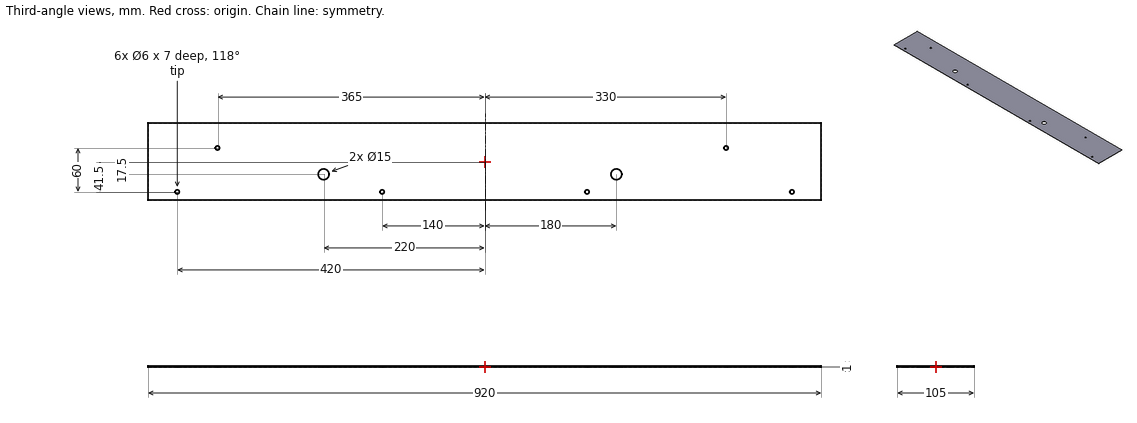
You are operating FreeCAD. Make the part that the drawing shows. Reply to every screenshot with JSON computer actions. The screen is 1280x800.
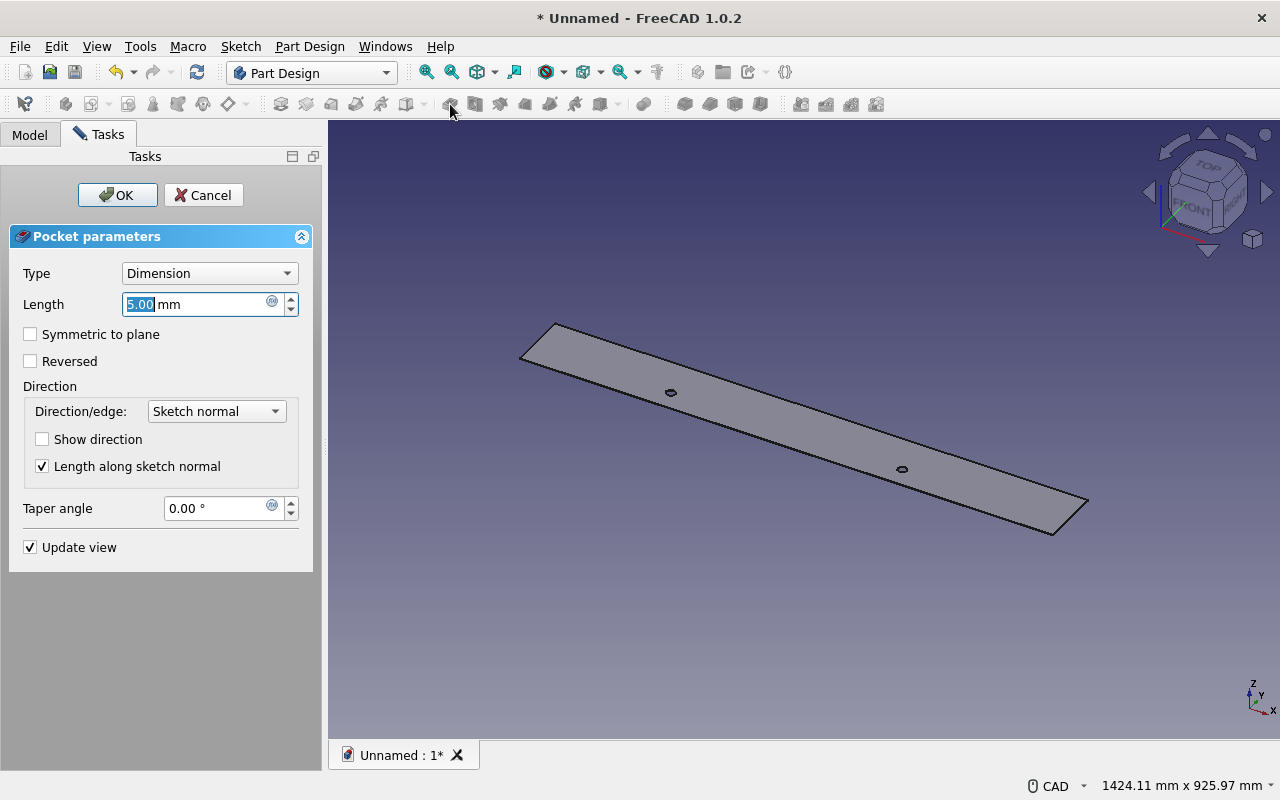
{"action": "left_click", "coordinate": [210, 274]}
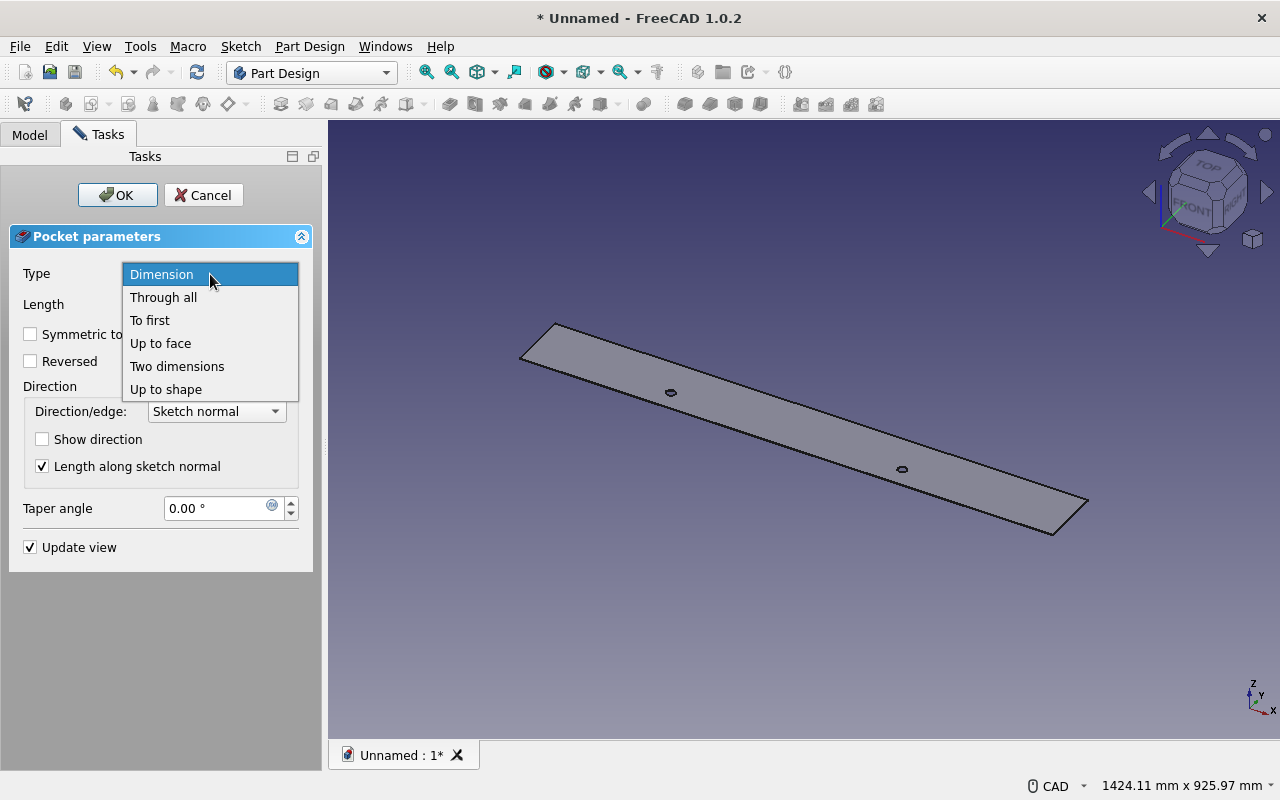
{"action": "left_click", "coordinate": [208, 298]}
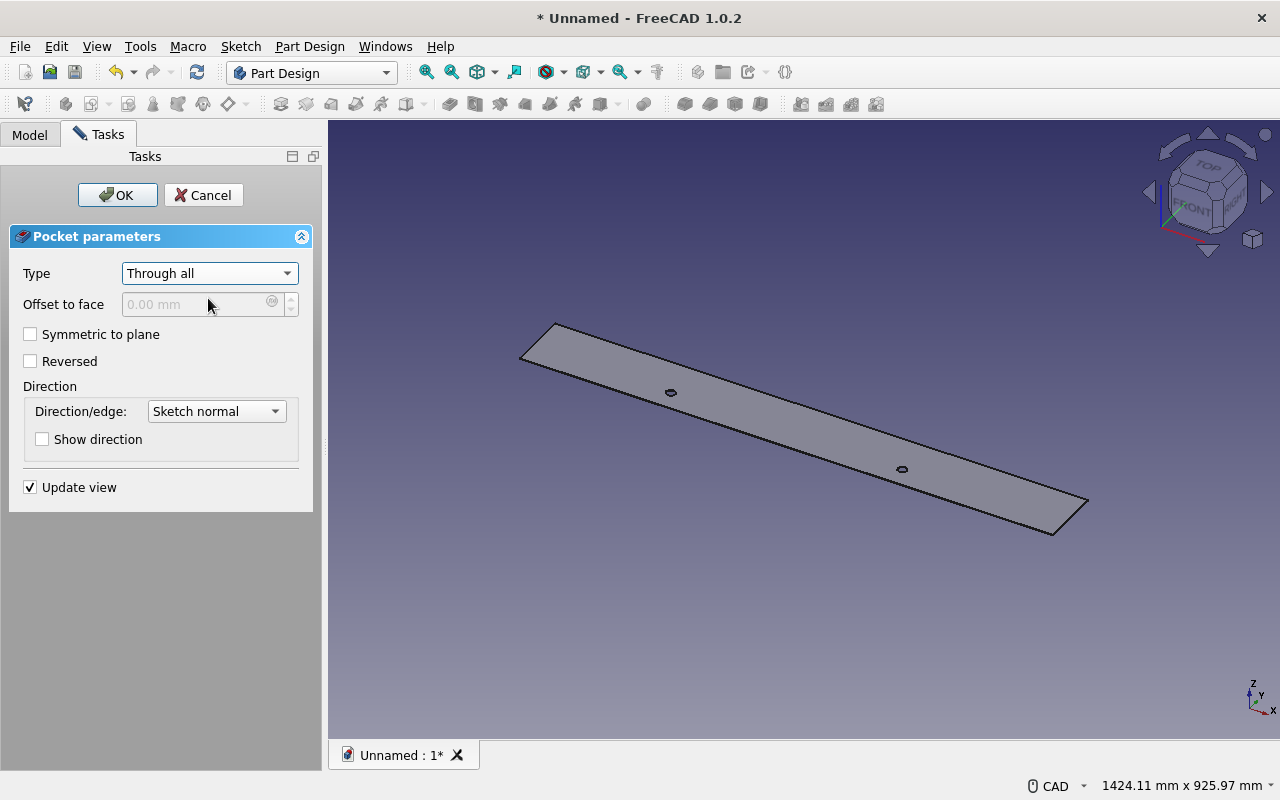
{"action": "left_click", "coordinate": [118, 195]}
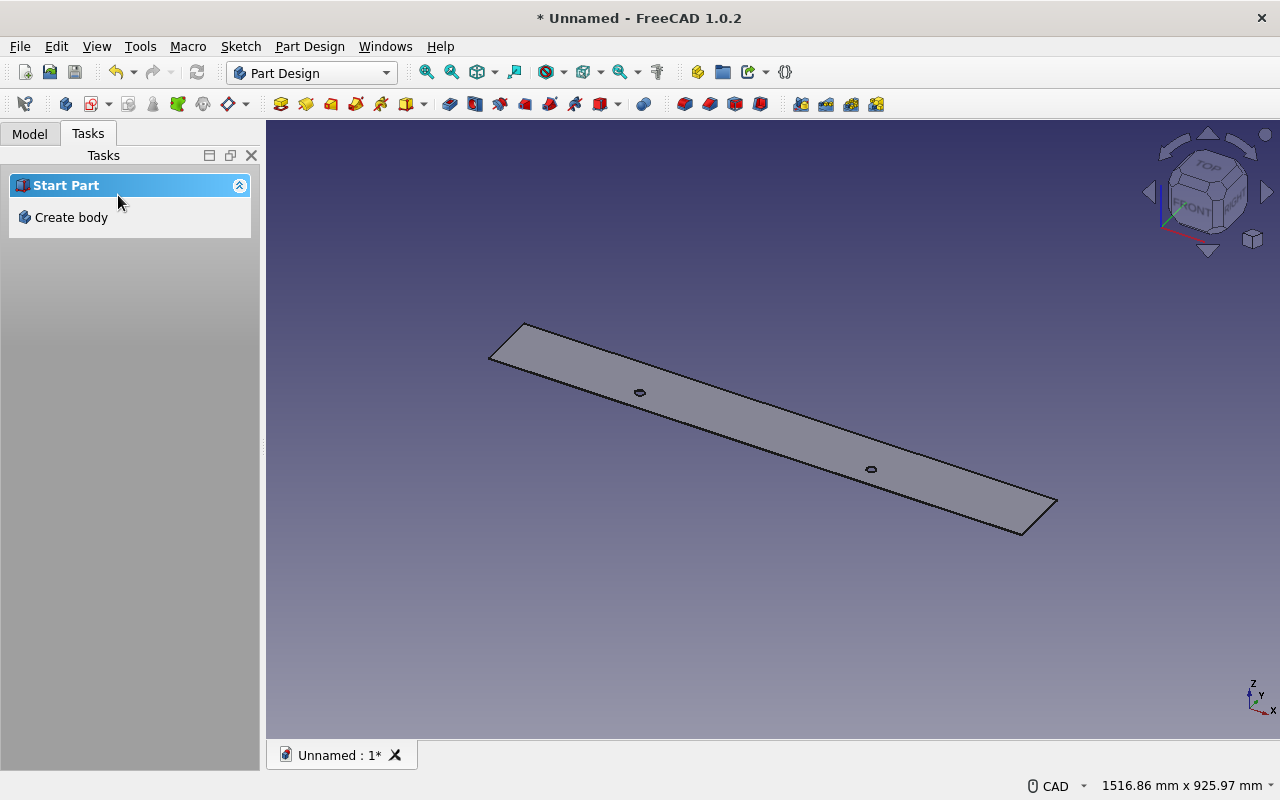
{"action": "left_click", "coordinate": [1001, 504]}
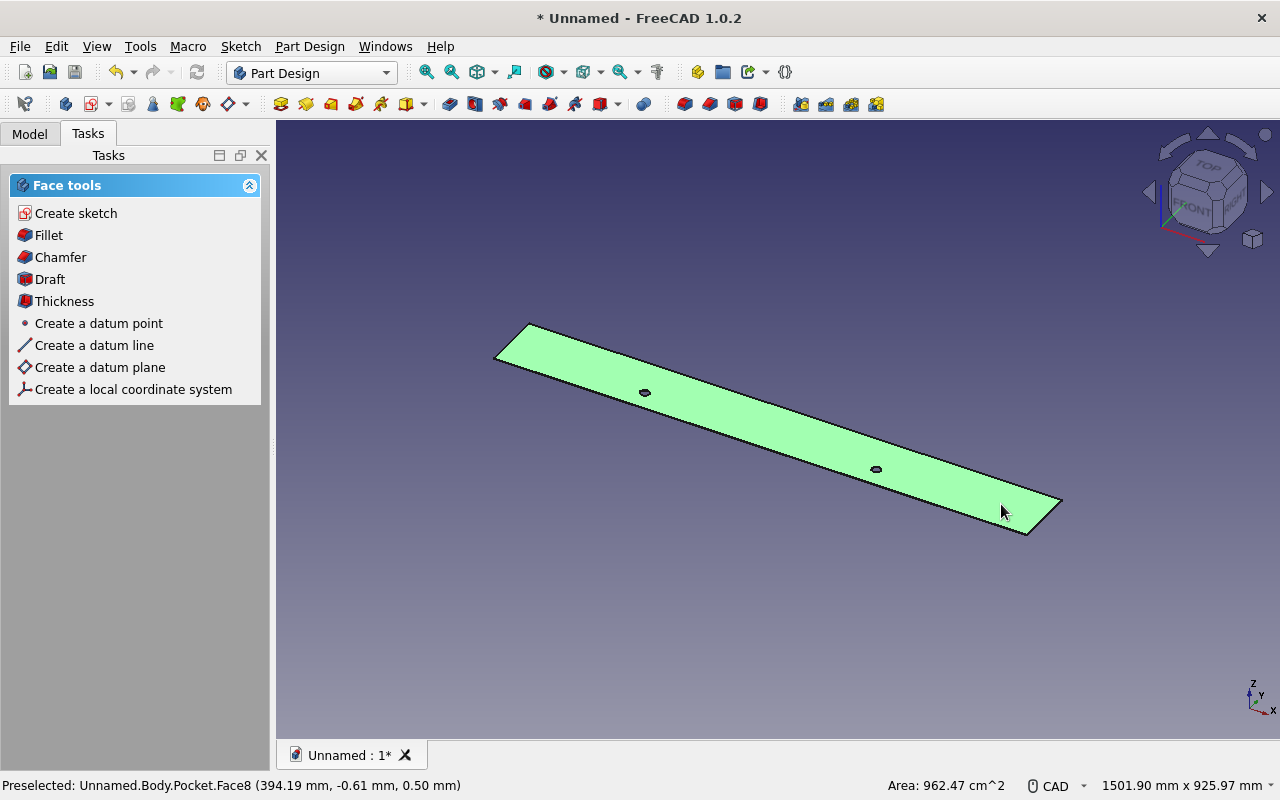
{"action": "left_click", "coordinate": [90, 104]}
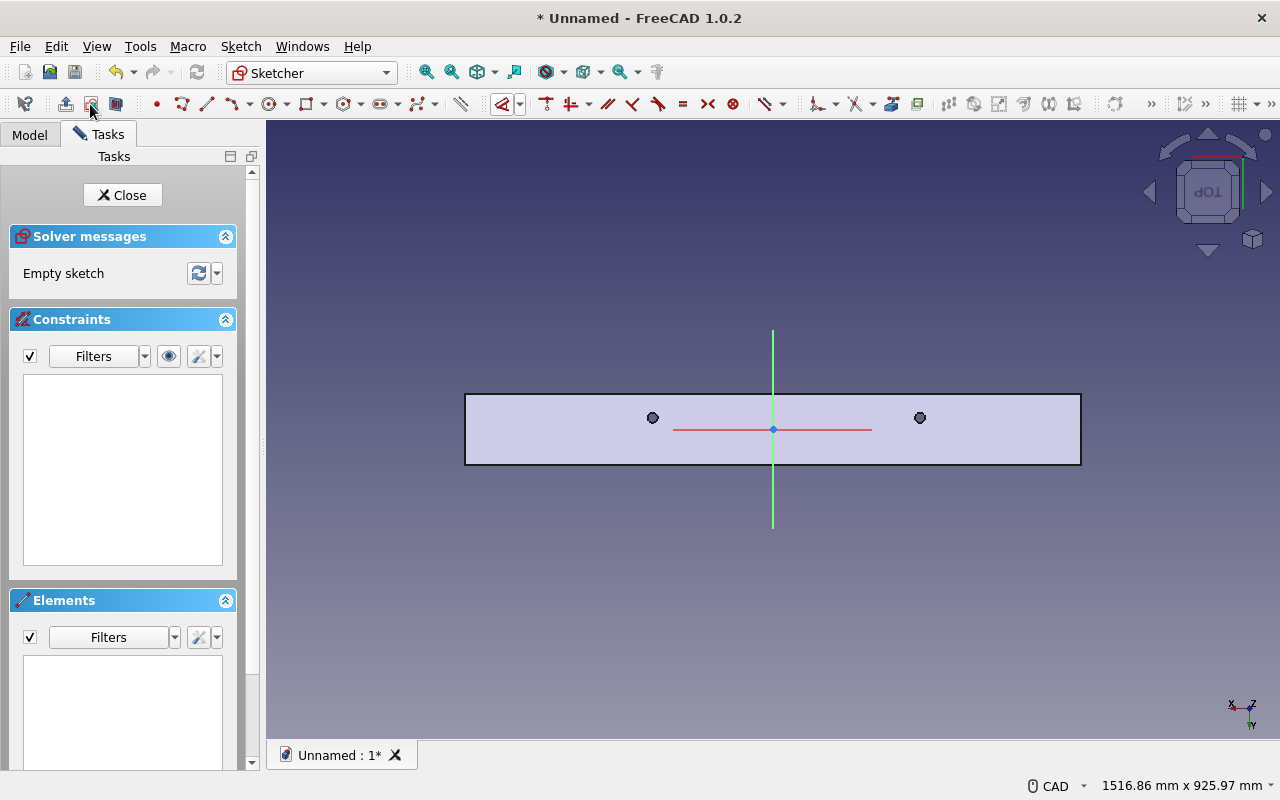
{"action": "left_click", "coordinate": [268, 104]}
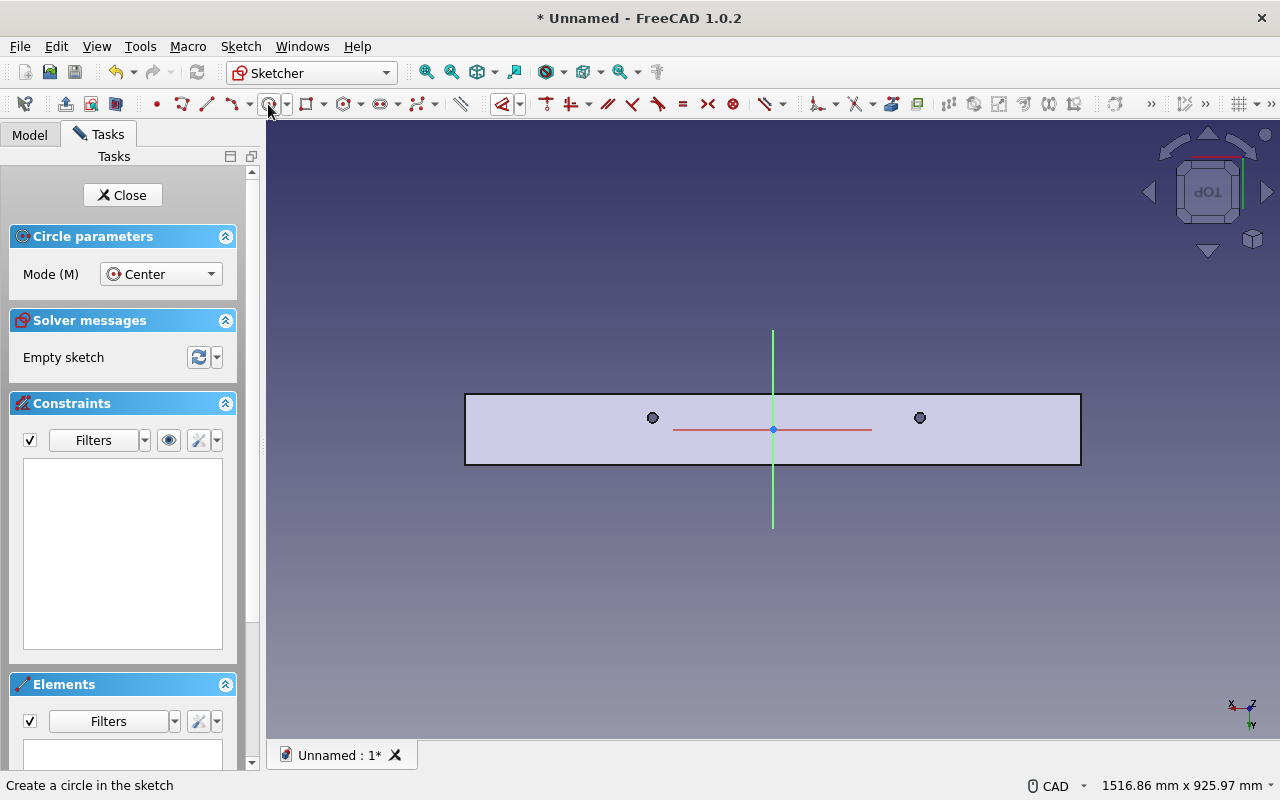
{"action": "scroll", "coordinate": [1054, 402], "scroll_direction": "up", "scroll_amount": 13}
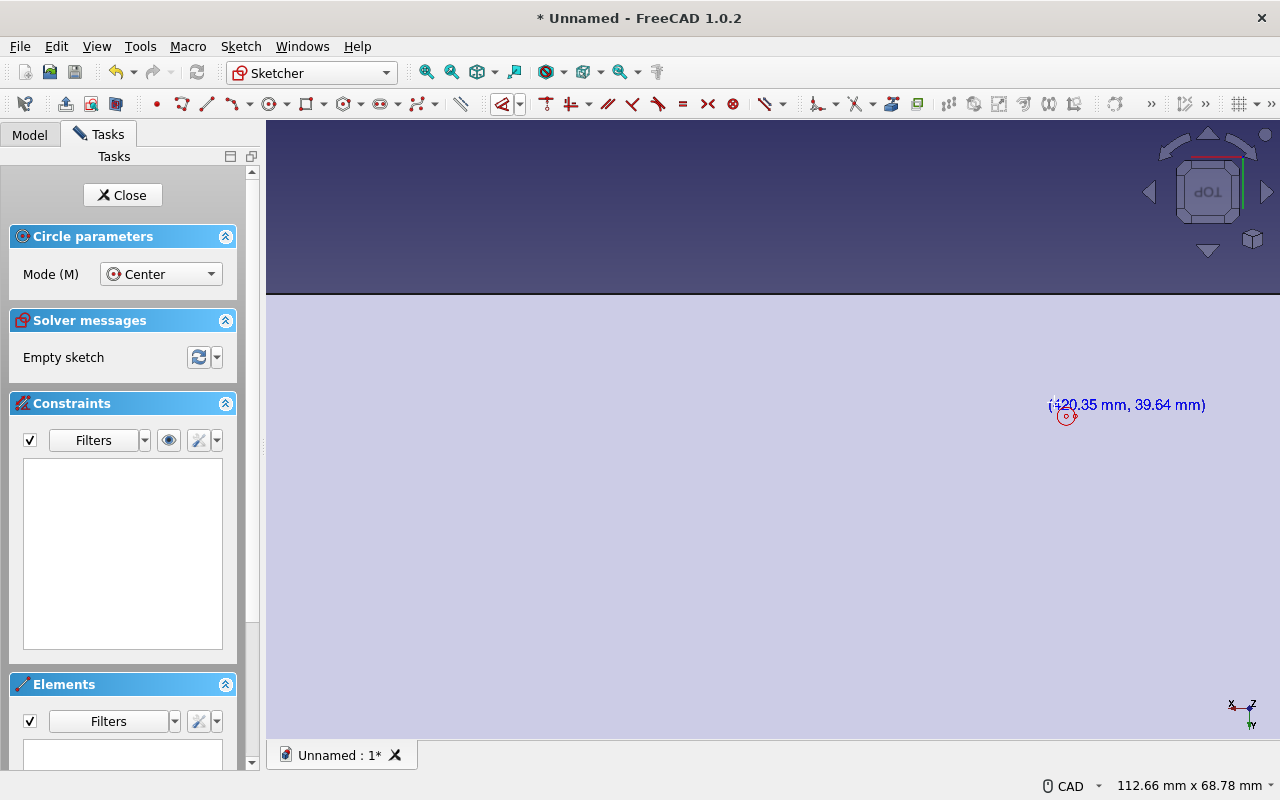
{"action": "scroll", "coordinate": [981, 411], "scroll_direction": "down", "scroll_amount": 13}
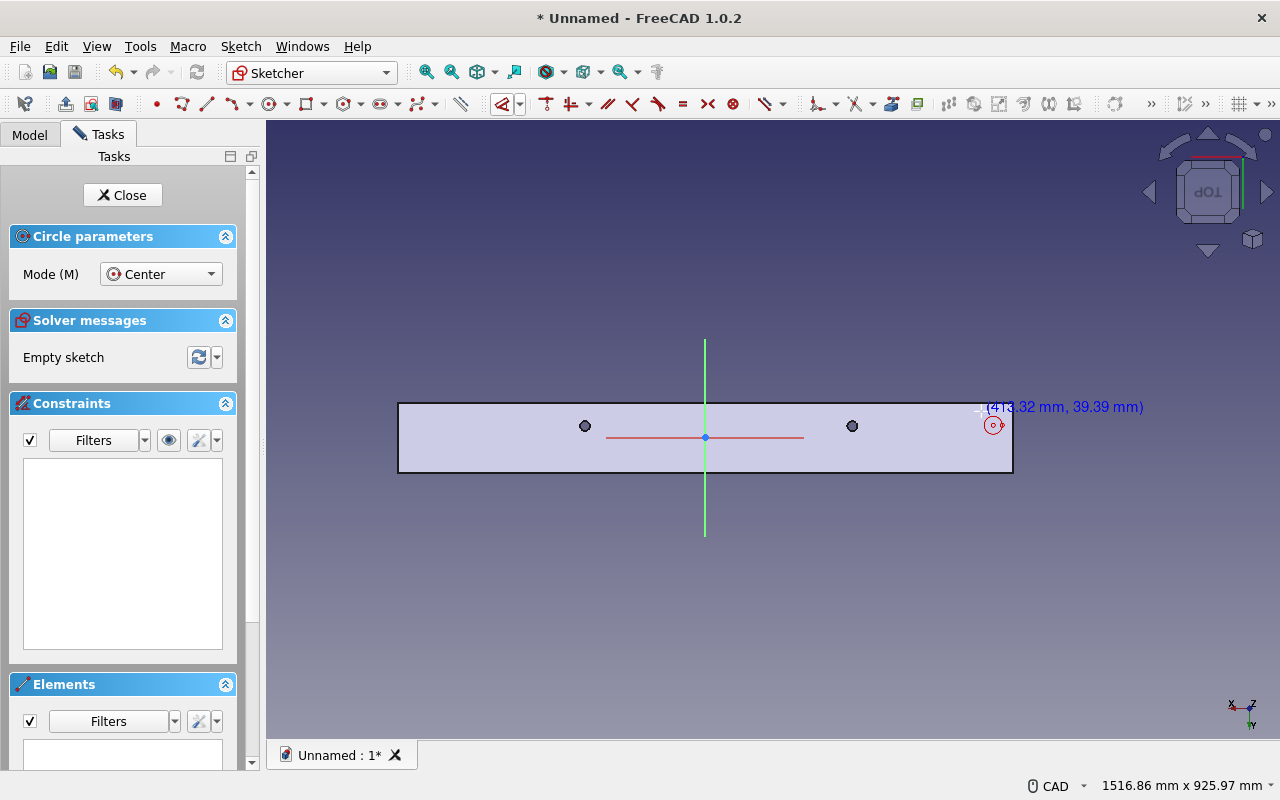
{"action": "left_click", "coordinate": [986, 410]}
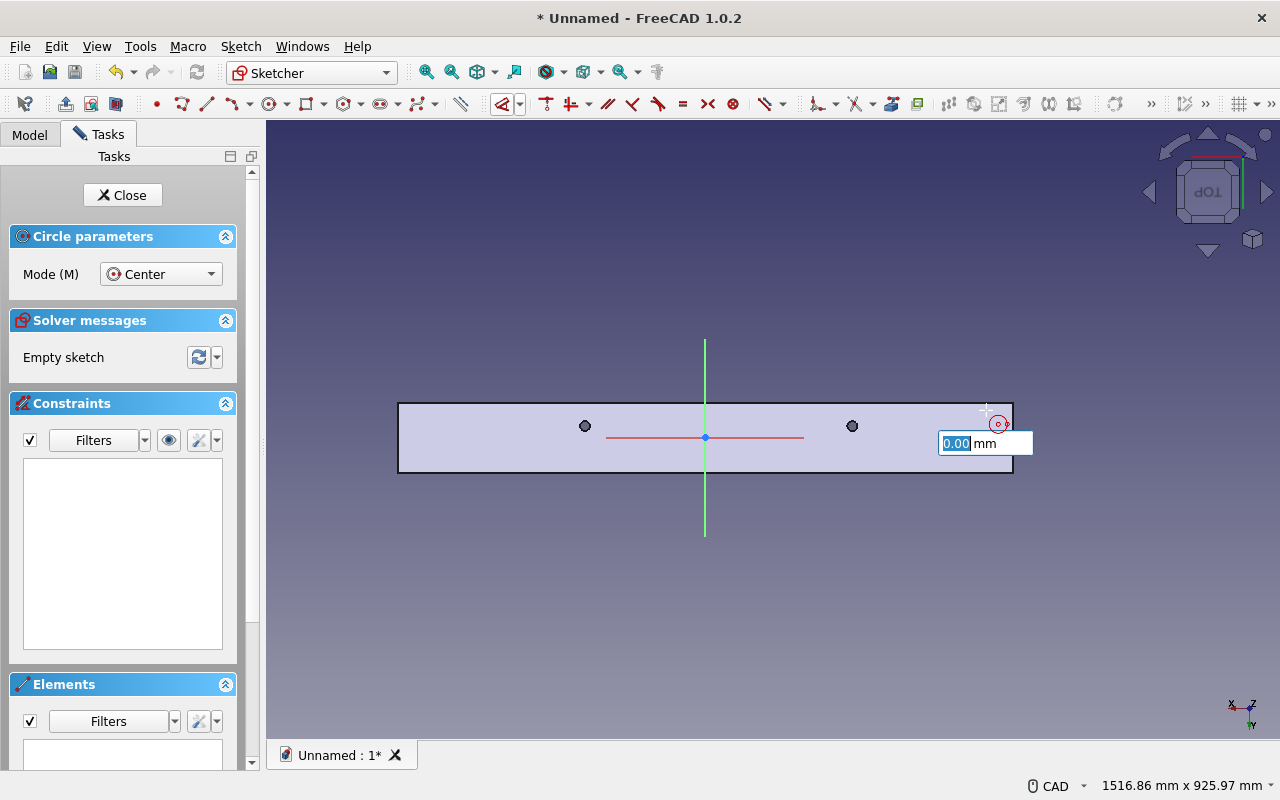
{"action": "scroll", "coordinate": [988, 409], "scroll_direction": "up", "scroll_amount": 11}